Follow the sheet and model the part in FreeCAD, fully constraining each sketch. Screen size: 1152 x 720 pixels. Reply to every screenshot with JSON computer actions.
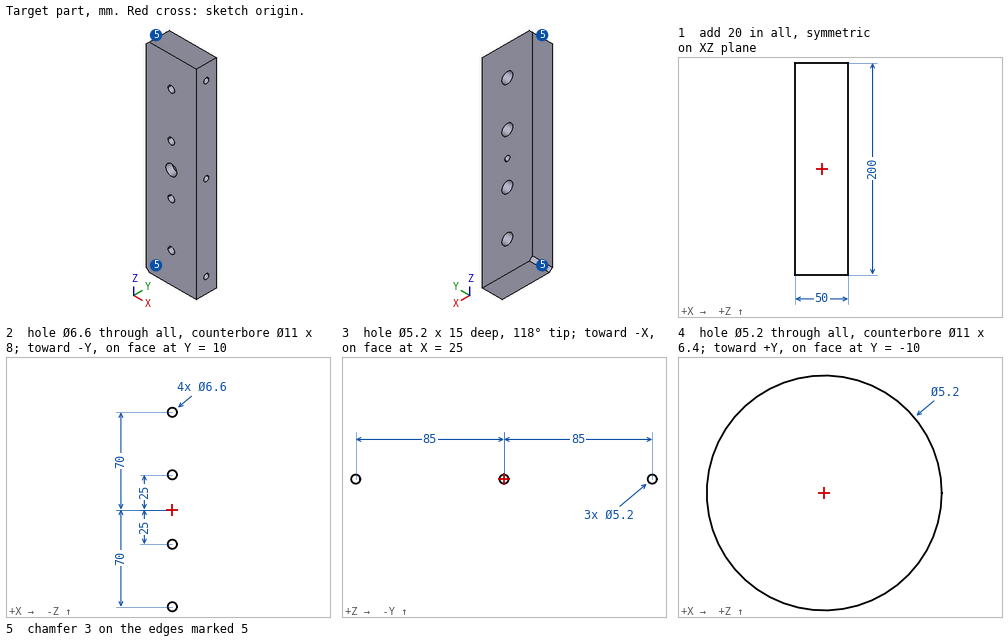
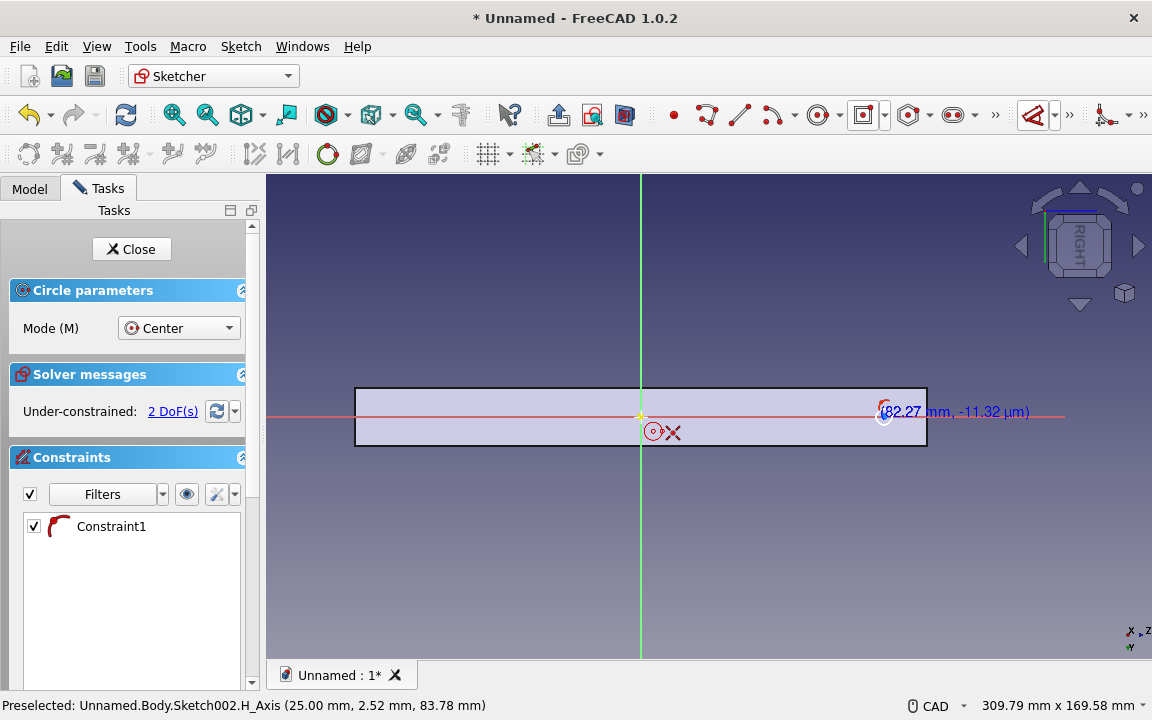
{"action": "left_click", "coordinate": [641, 417]}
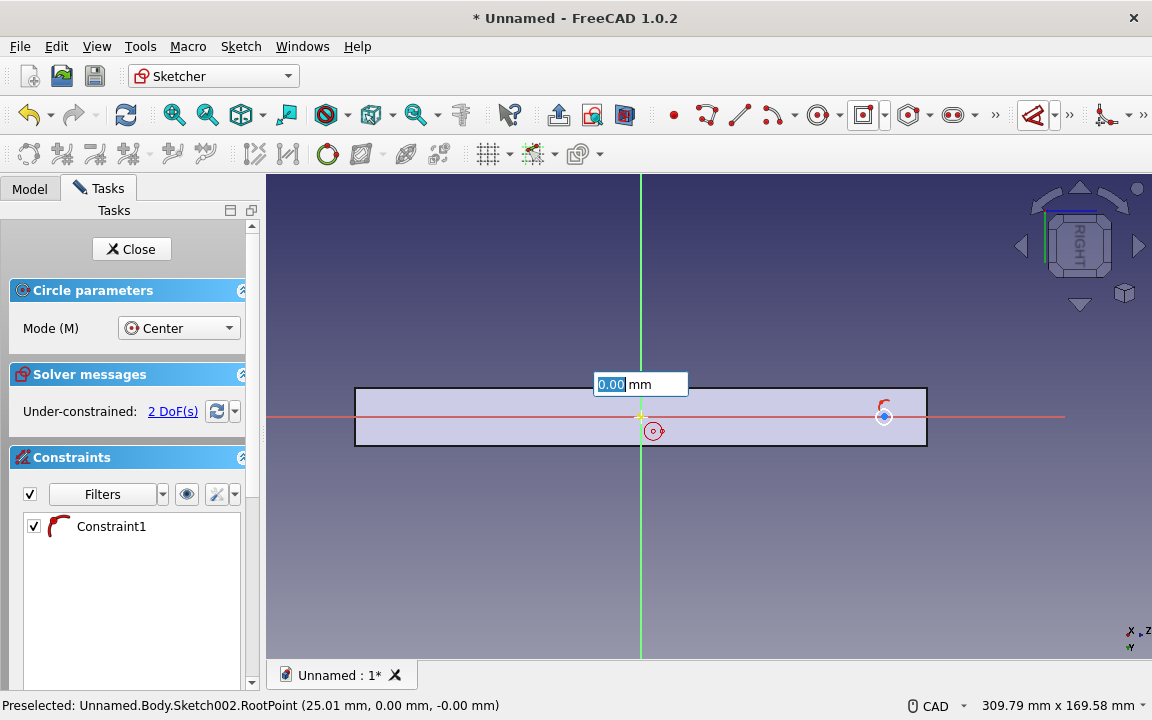
{"action": "scroll", "coordinate": [646, 412], "scroll_direction": "up", "scroll_amount": 6}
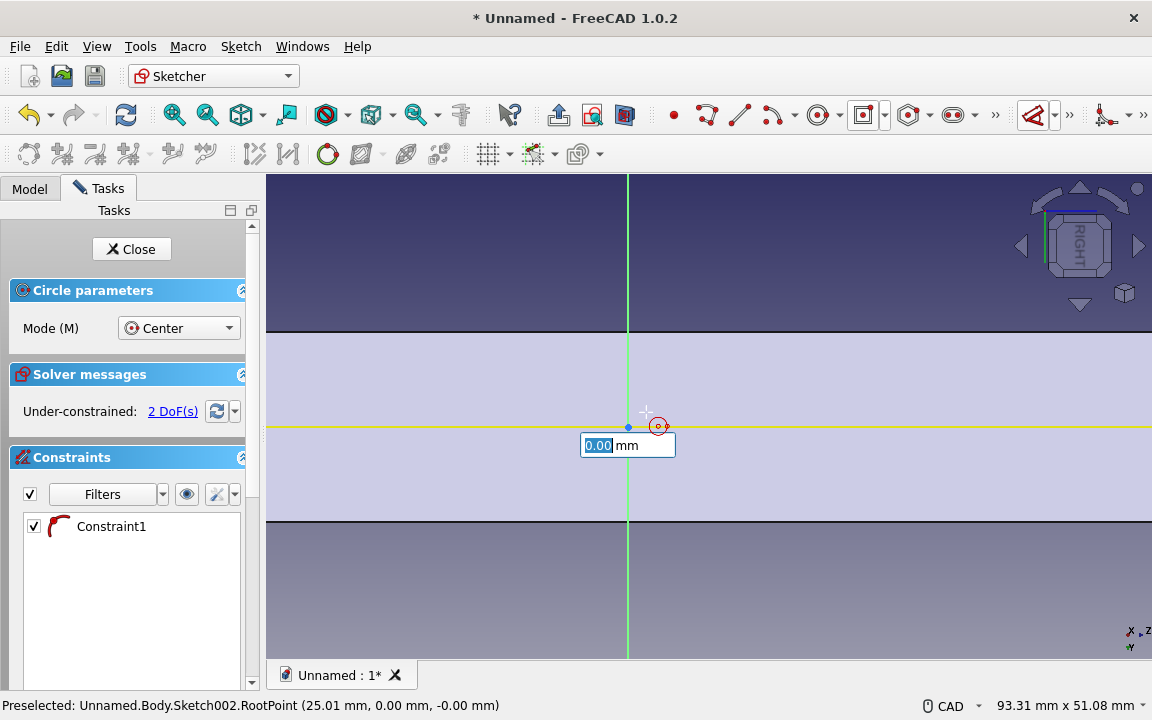
{"action": "left_click", "coordinate": [646, 410]}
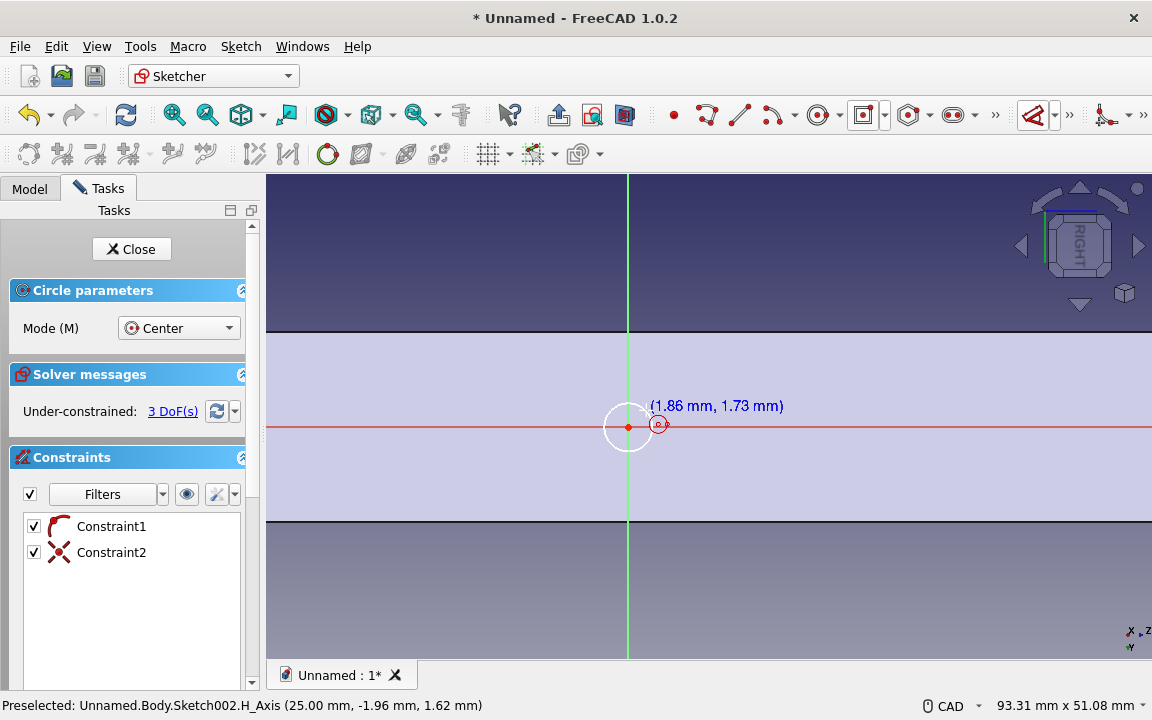
{"action": "scroll", "coordinate": [646, 412], "scroll_direction": "down", "scroll_amount": 6}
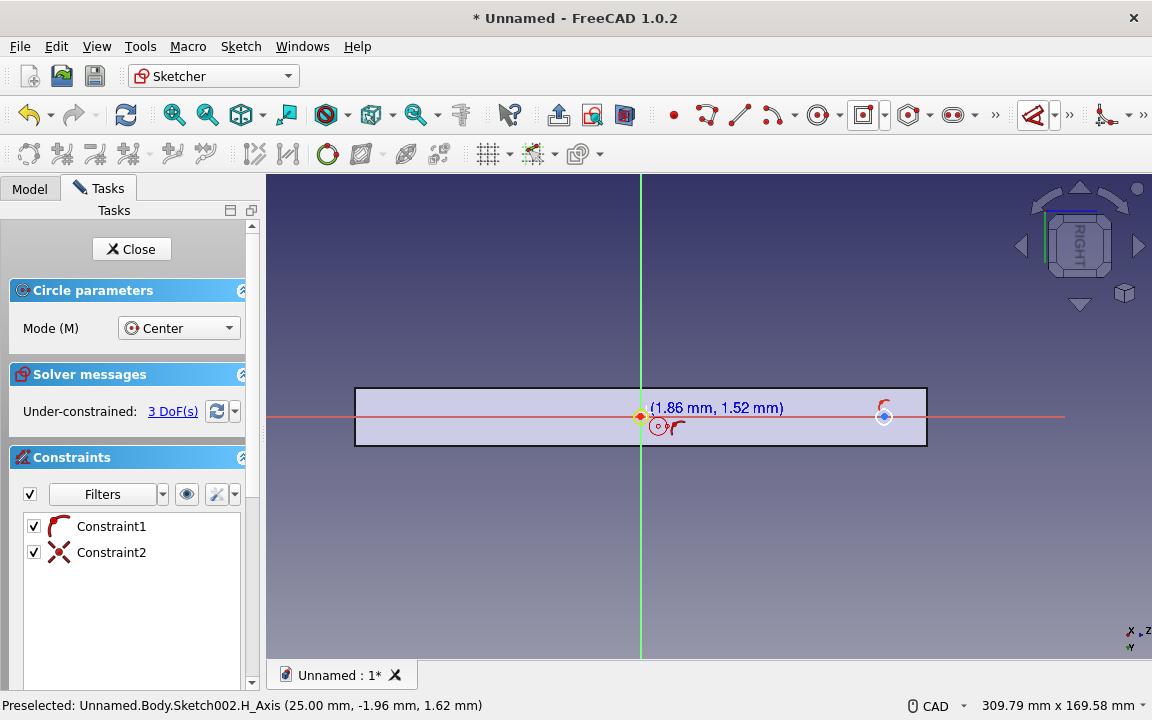
{"action": "scroll", "coordinate": [398, 417], "scroll_direction": "up", "scroll_amount": 6}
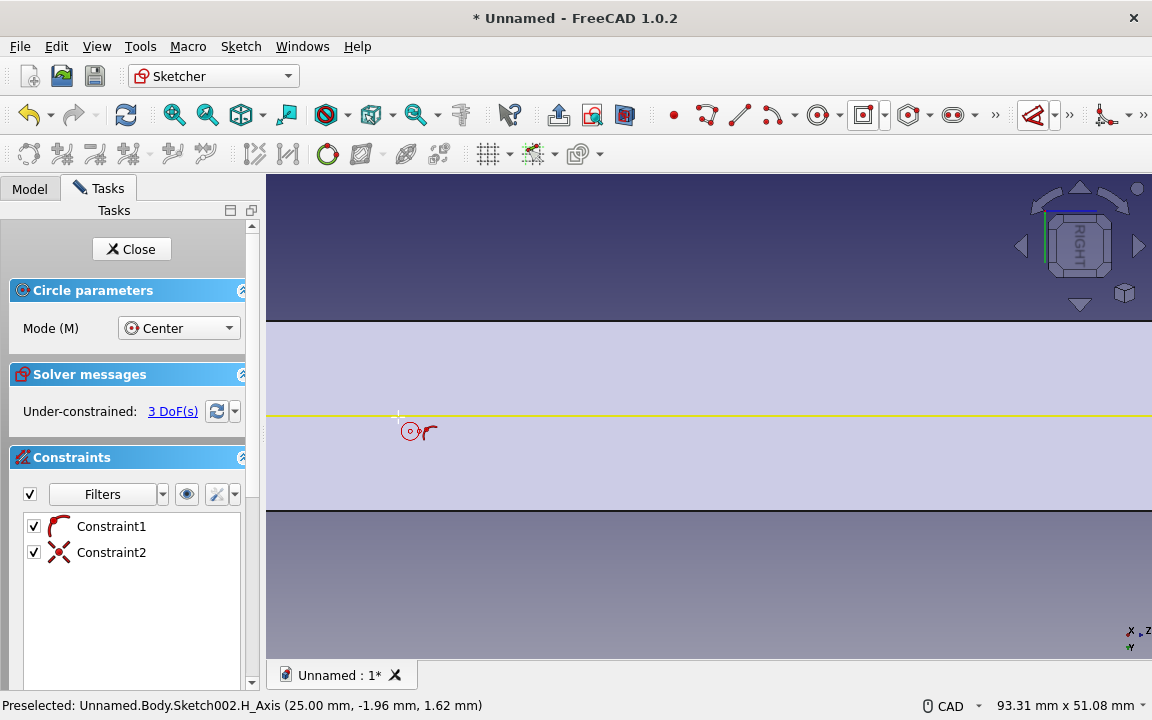
{"action": "scroll", "coordinate": [397, 417], "scroll_direction": "down", "scroll_amount": 6}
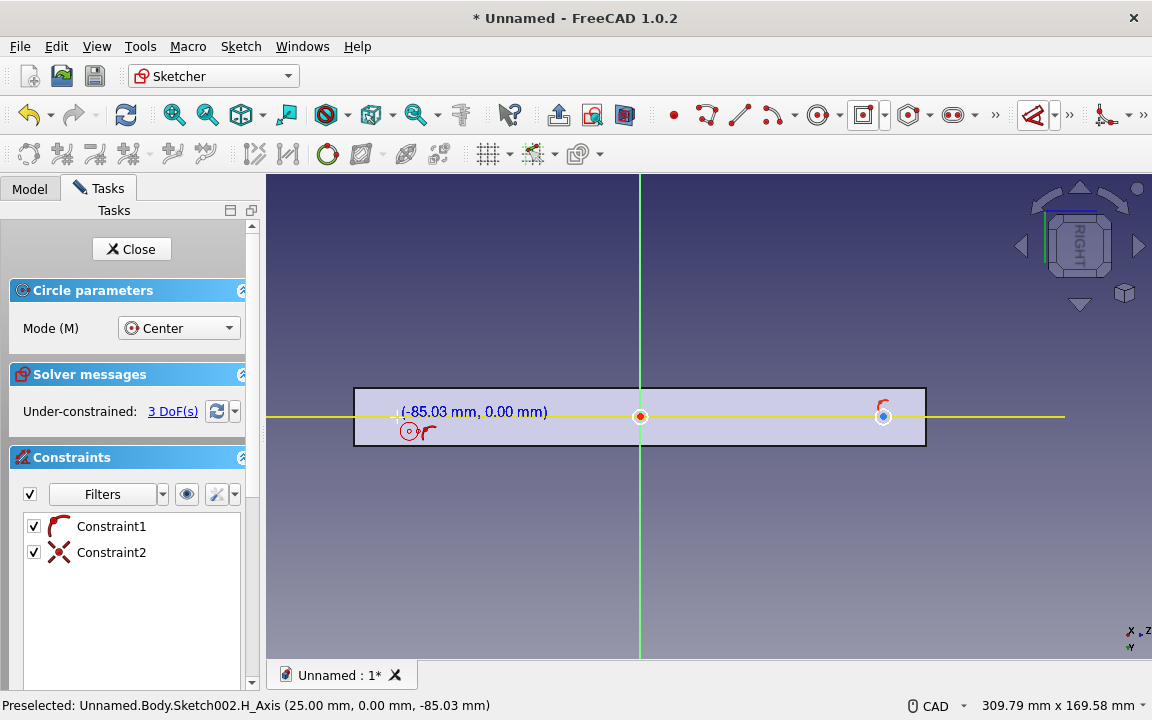
{"action": "left_click", "coordinate": [397, 417]}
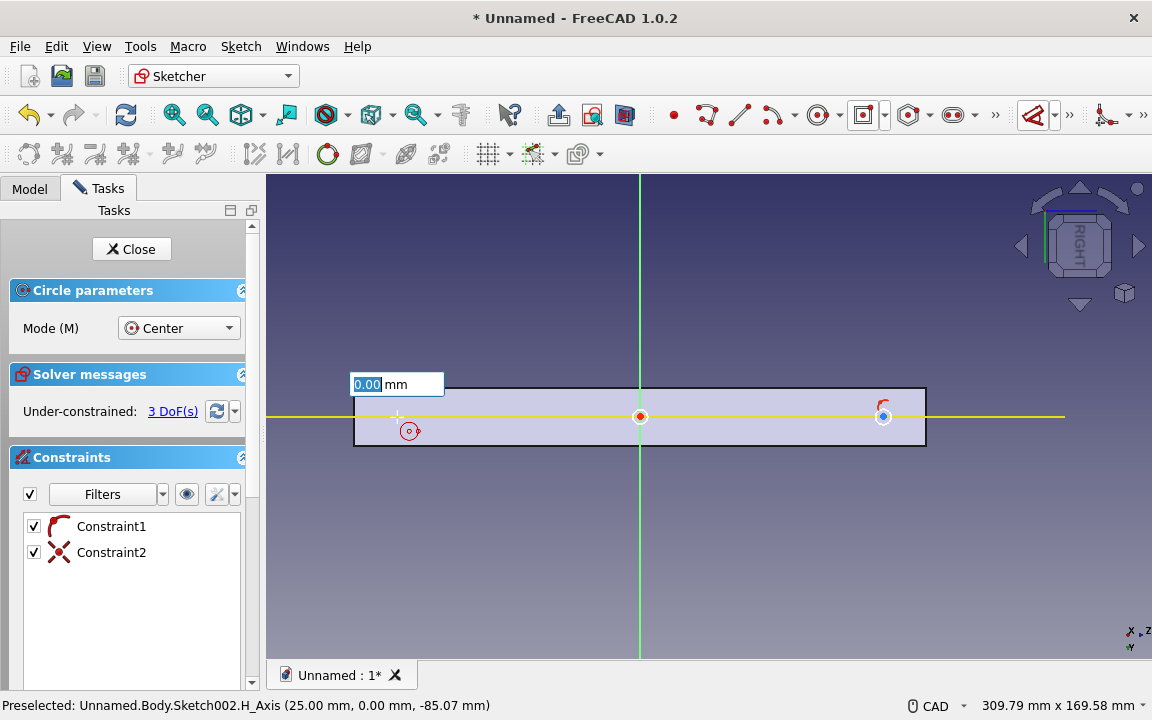
{"action": "scroll", "coordinate": [395, 424], "scroll_direction": "up", "scroll_amount": 5}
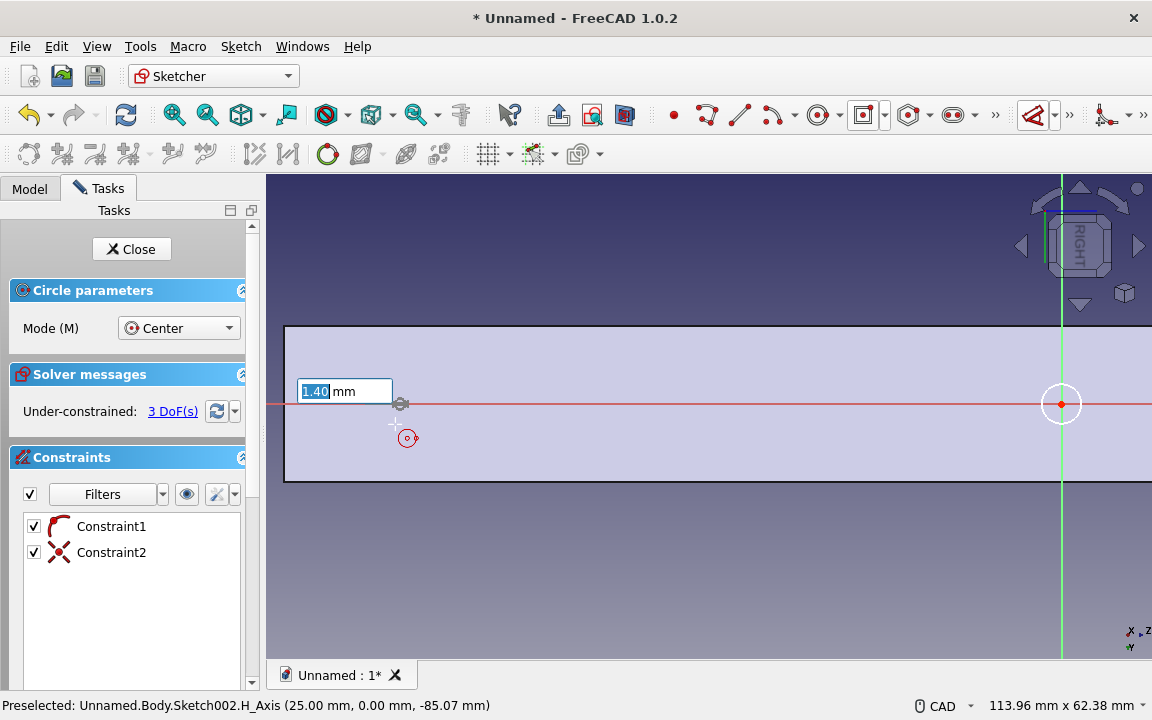
{"action": "left_click", "coordinate": [394, 423]}
{"action": "key", "text": "Escape"}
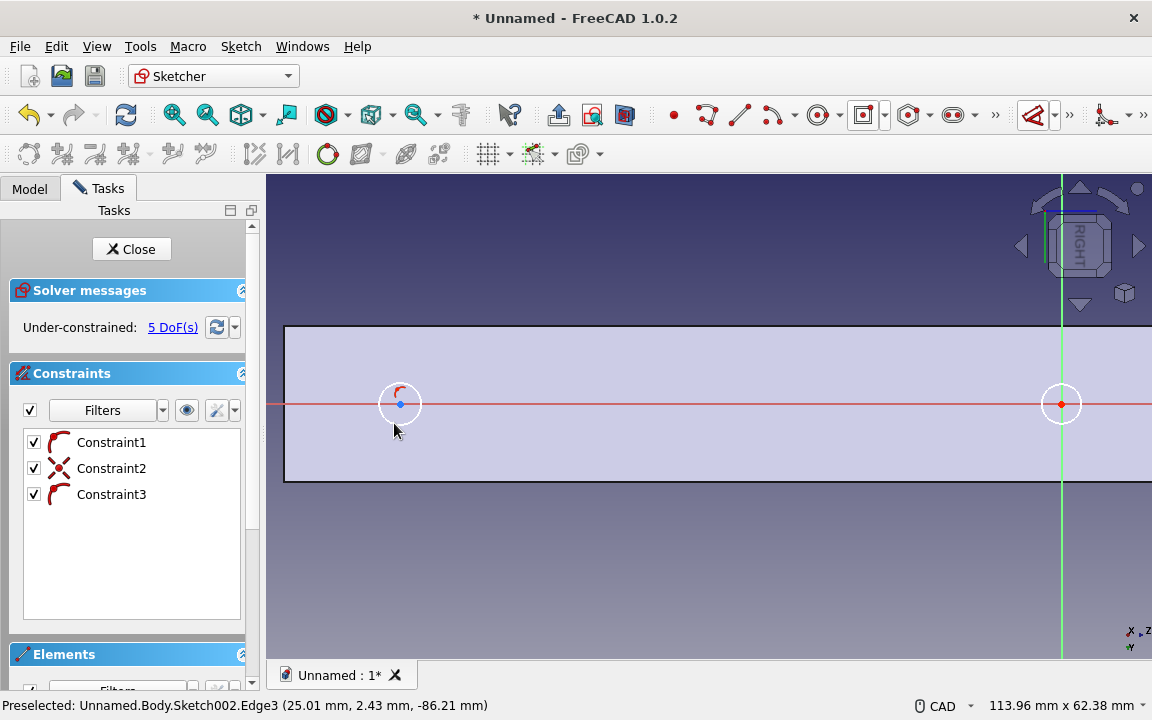
{"action": "scroll", "coordinate": [395, 424], "scroll_direction": "down", "scroll_amount": 5}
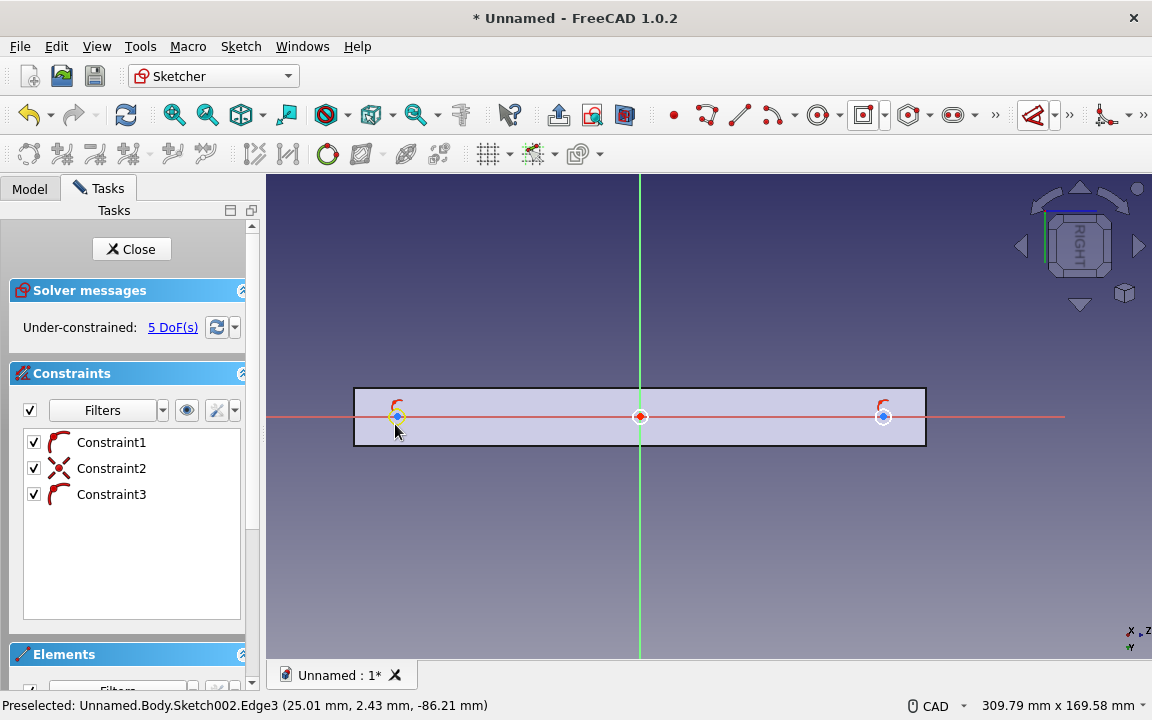
{"action": "scroll", "coordinate": [889, 412], "scroll_direction": "up", "scroll_amount": 5}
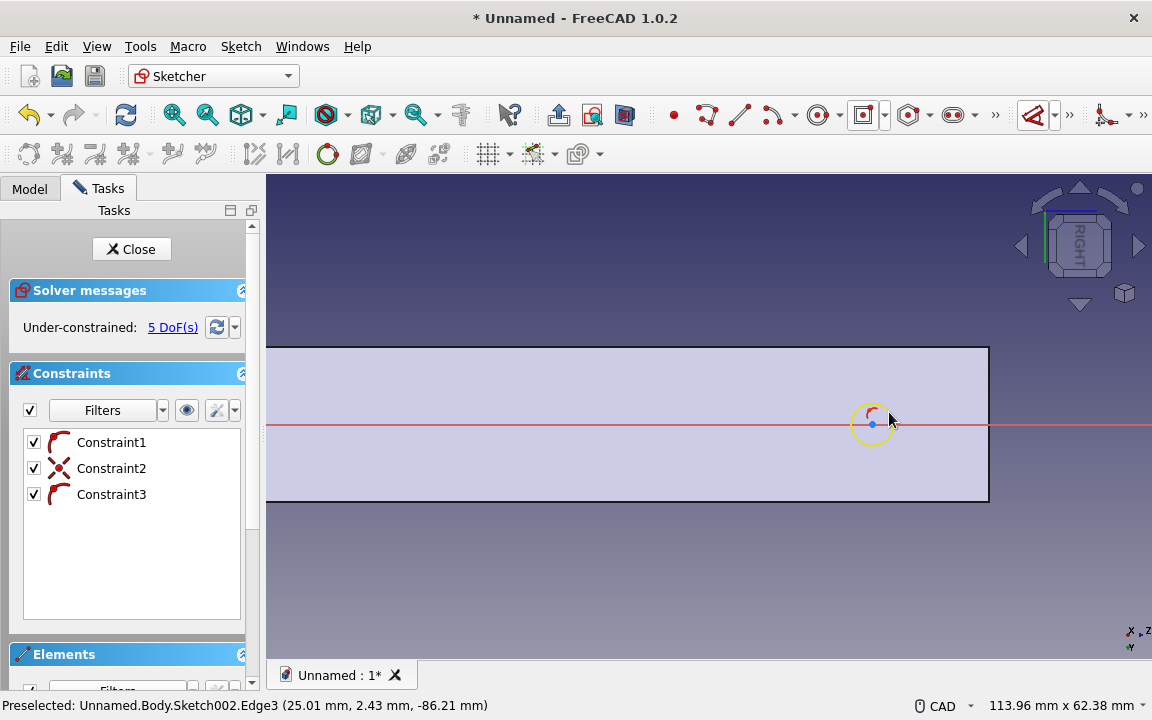
{"action": "left_click", "coordinate": [887, 410]}